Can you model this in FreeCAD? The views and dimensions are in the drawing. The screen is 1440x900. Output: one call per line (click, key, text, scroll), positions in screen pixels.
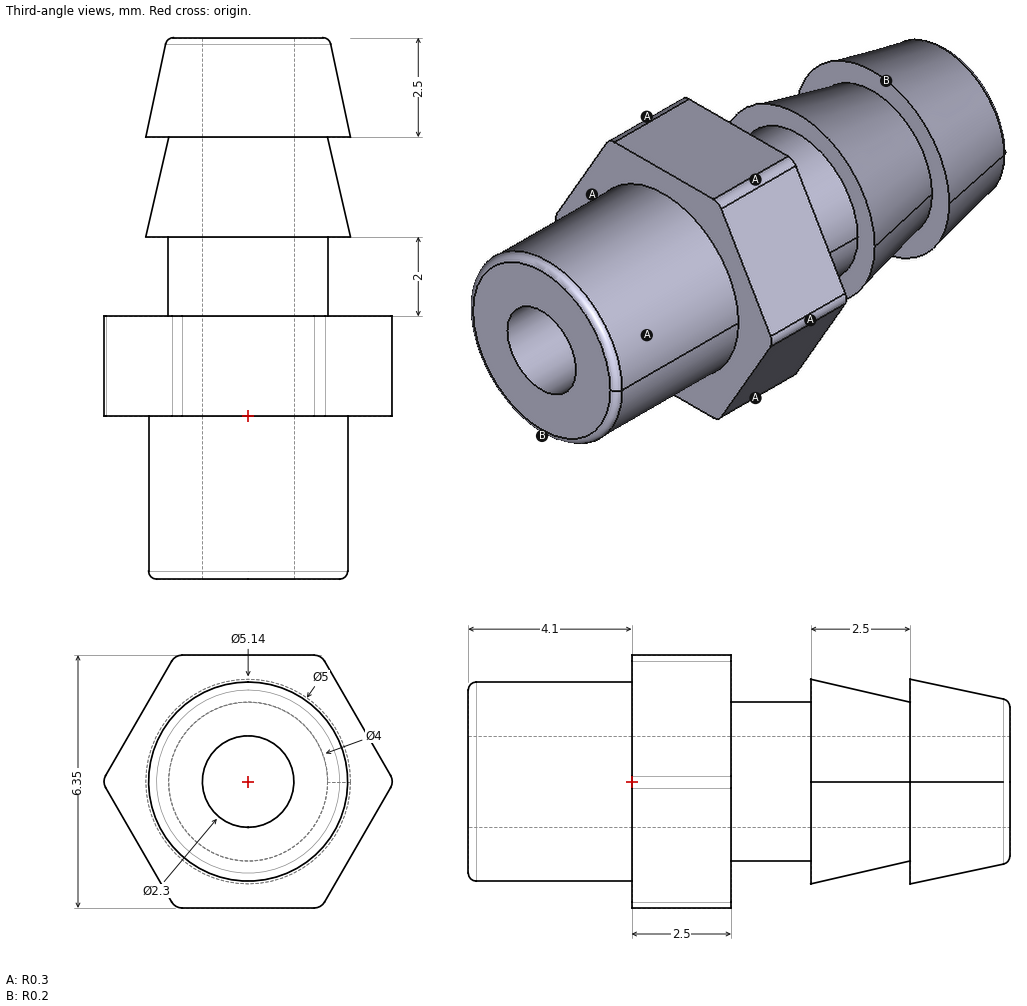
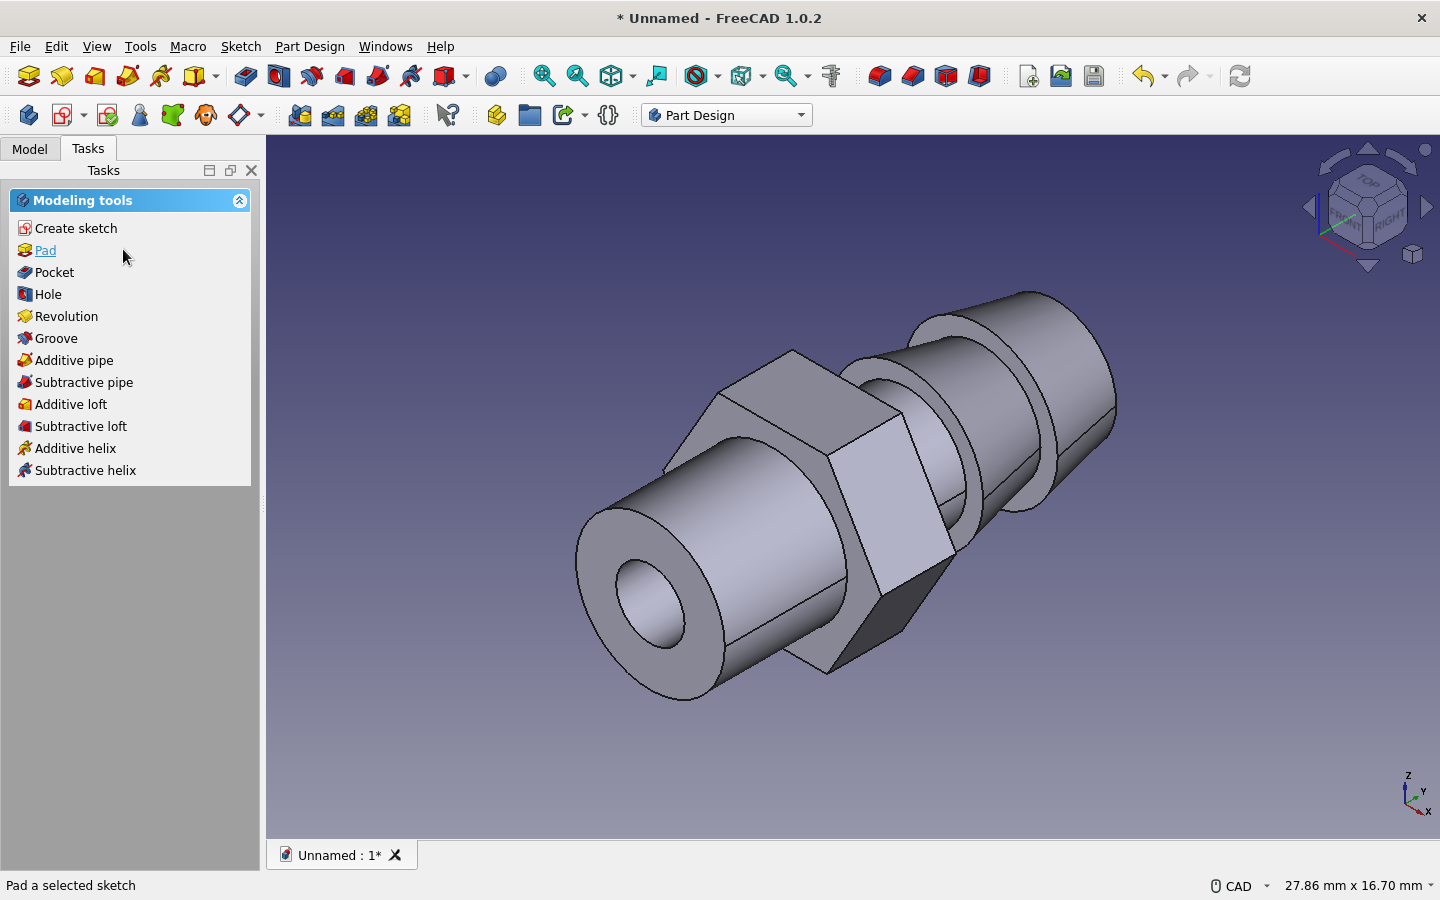
click(246, 76)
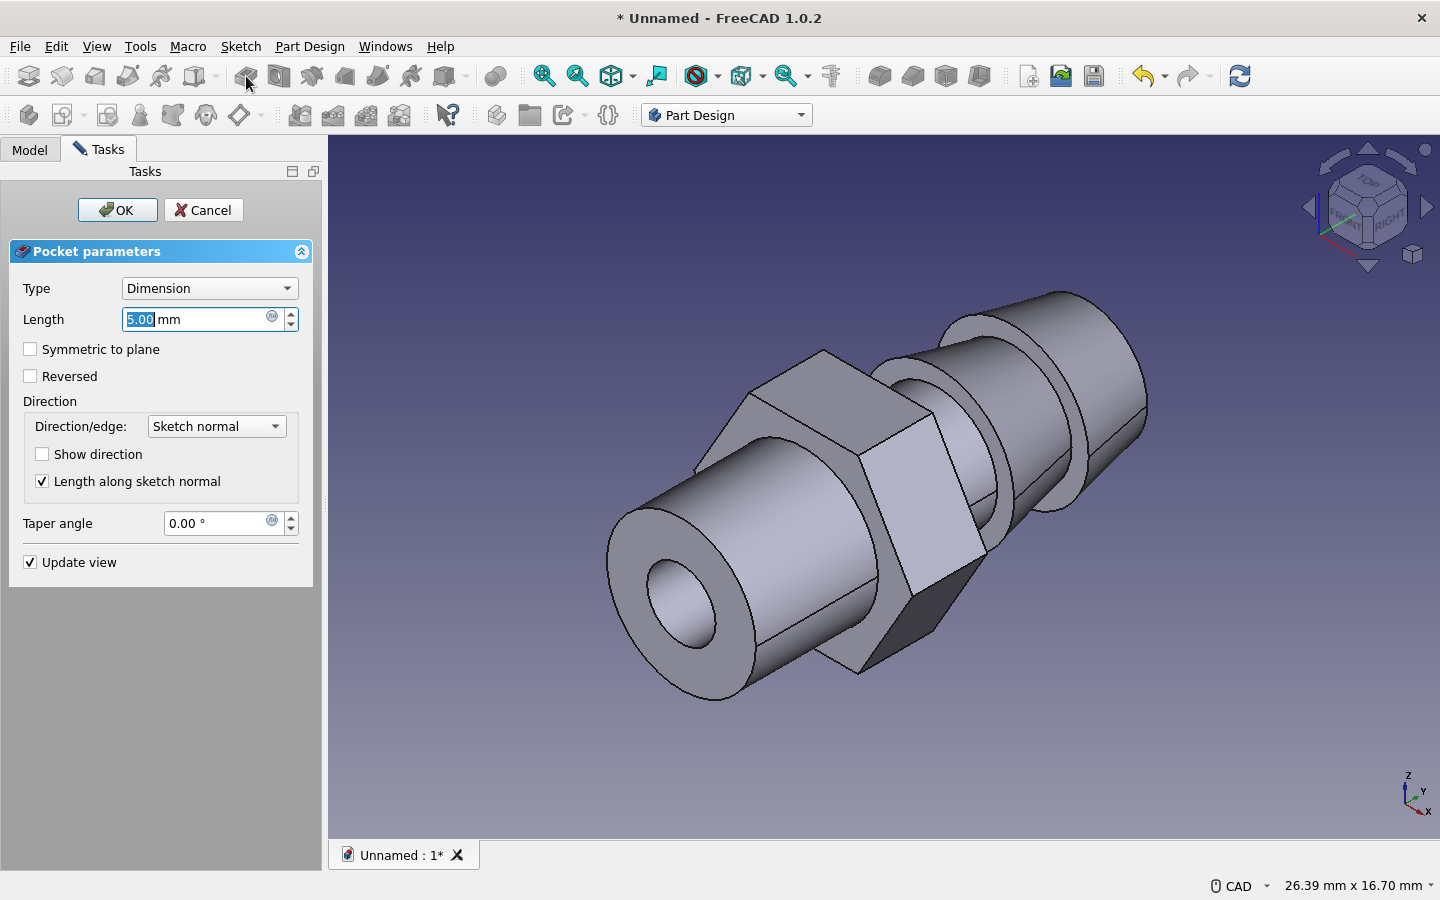
click(210, 288)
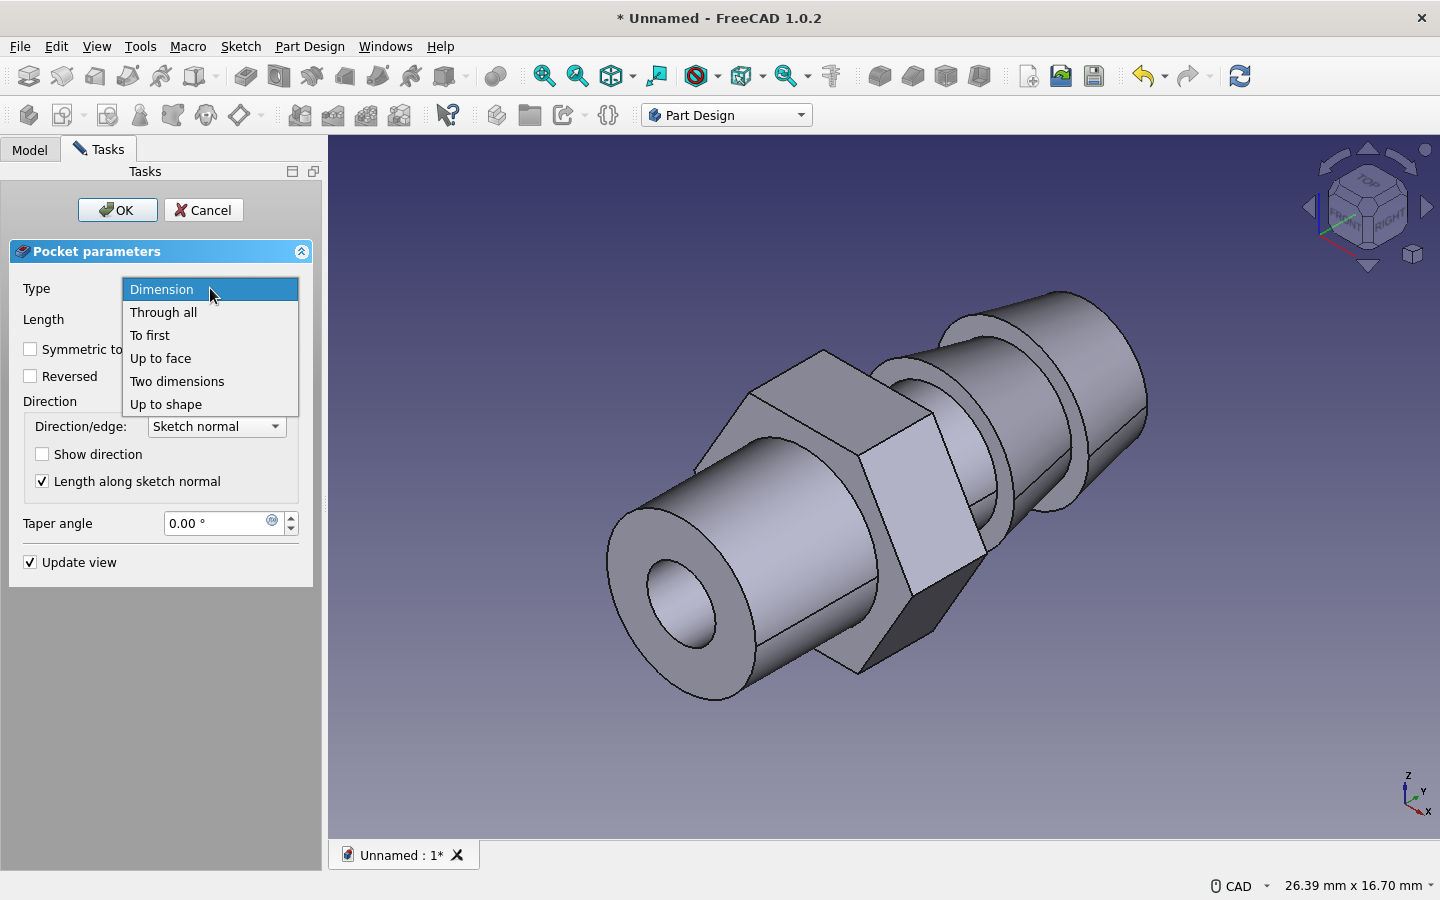
click(208, 312)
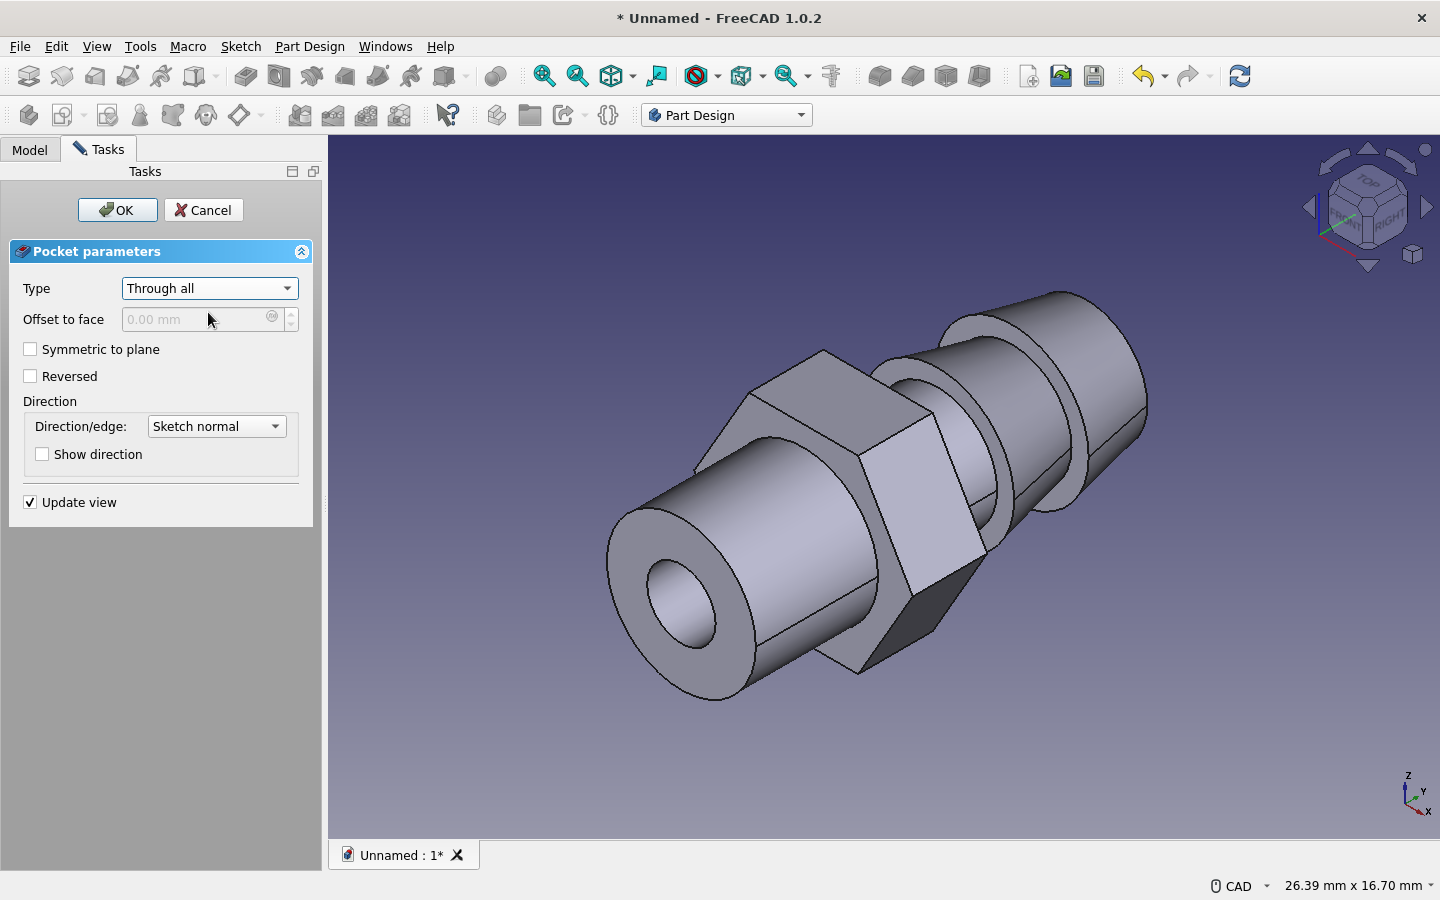
click(118, 210)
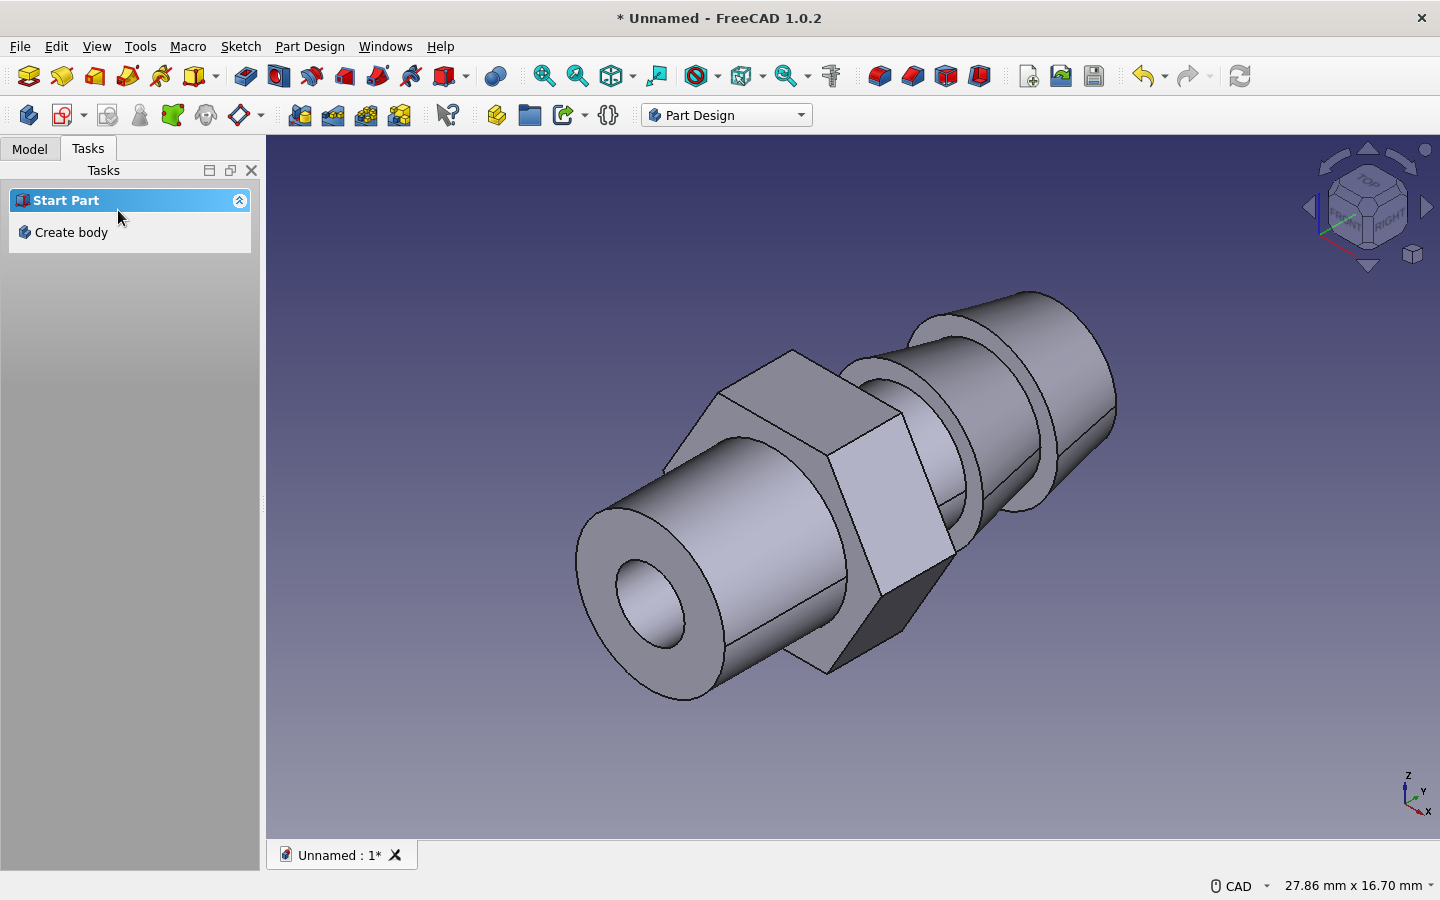
click(864, 433)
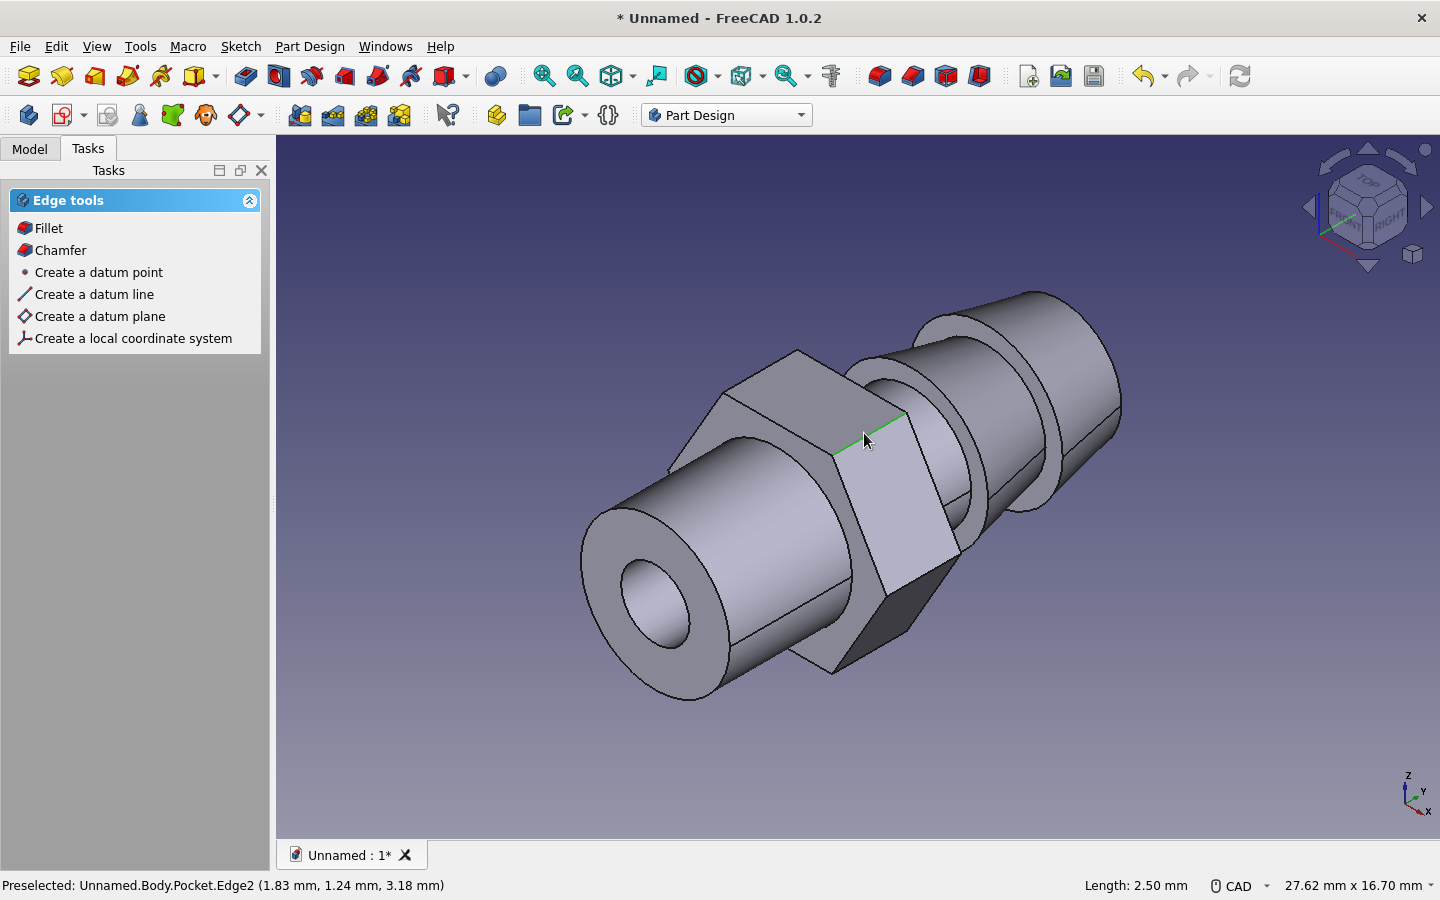
key(2)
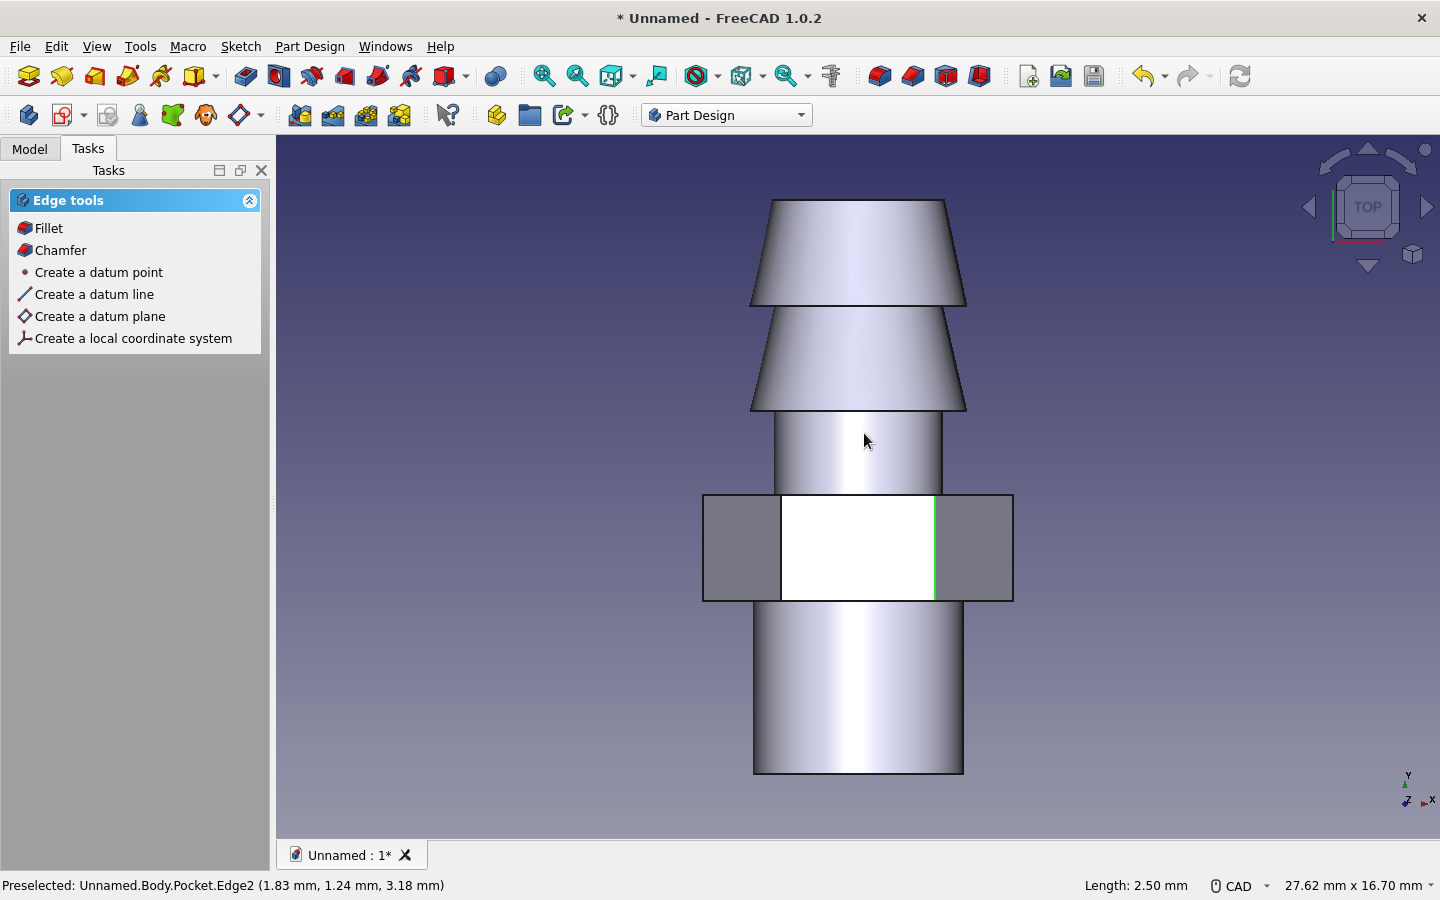
click(781, 547, ctrl)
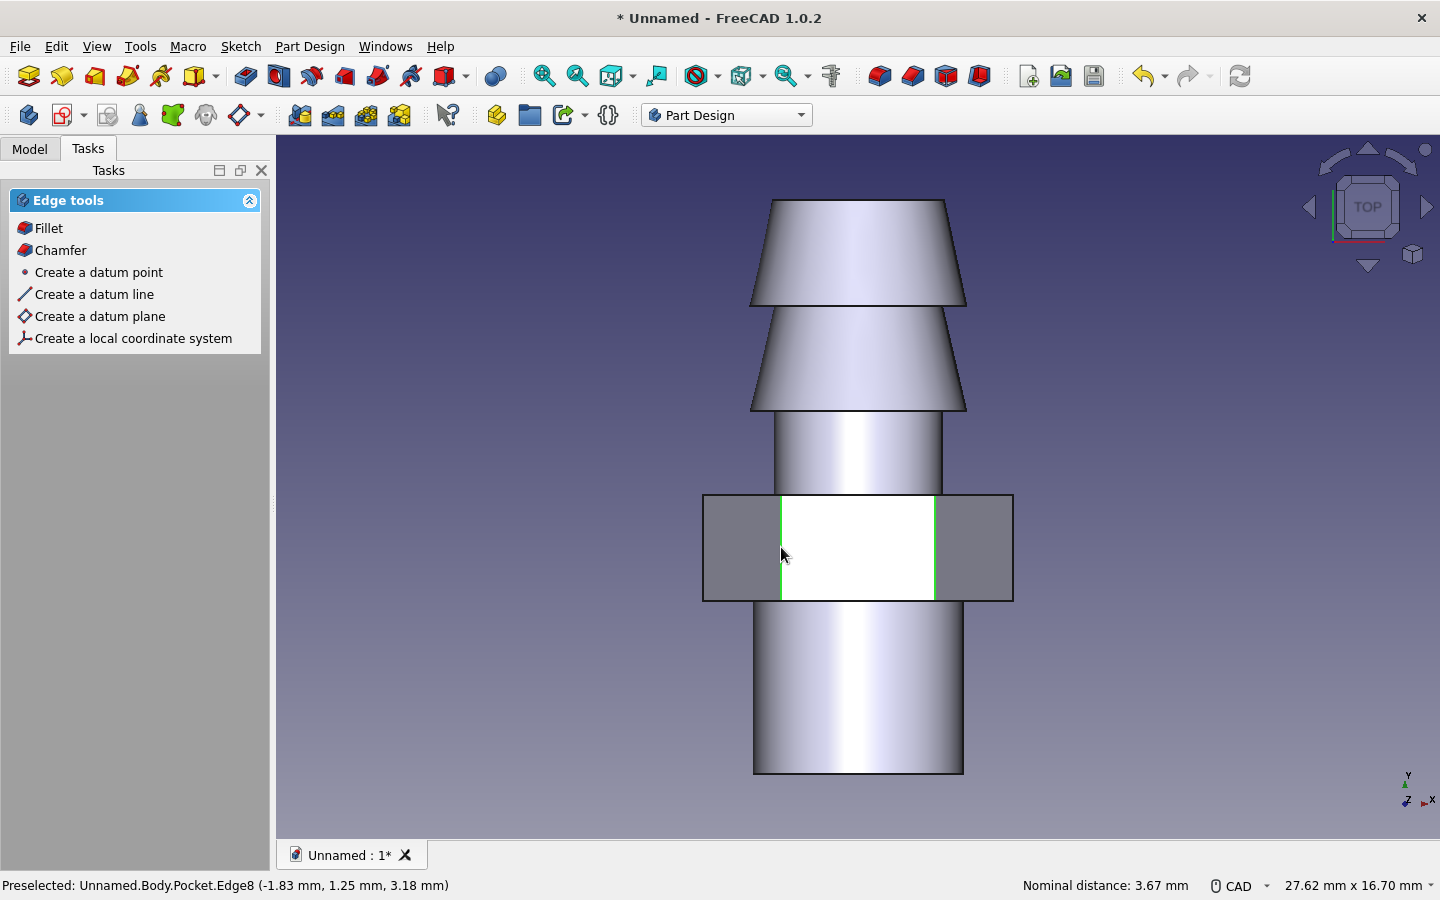
key(0)